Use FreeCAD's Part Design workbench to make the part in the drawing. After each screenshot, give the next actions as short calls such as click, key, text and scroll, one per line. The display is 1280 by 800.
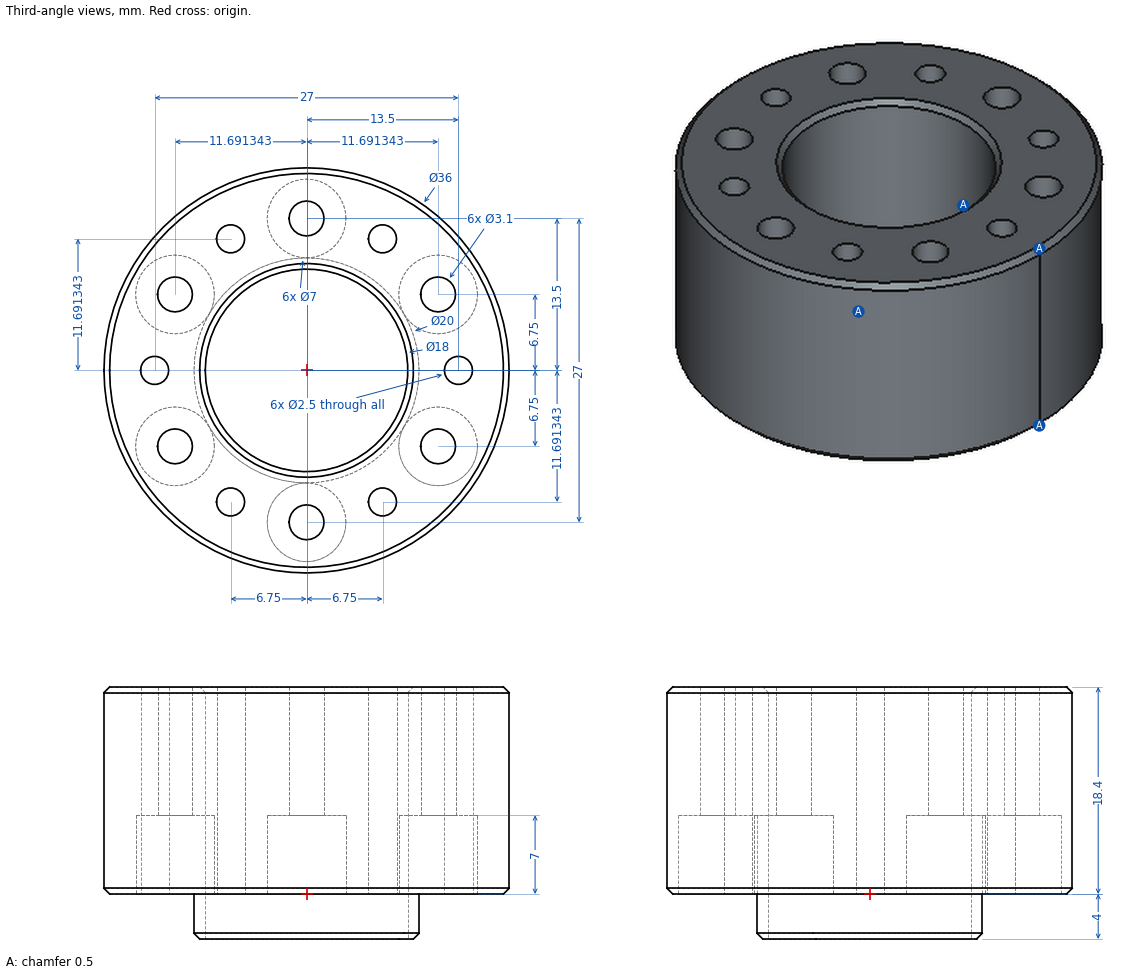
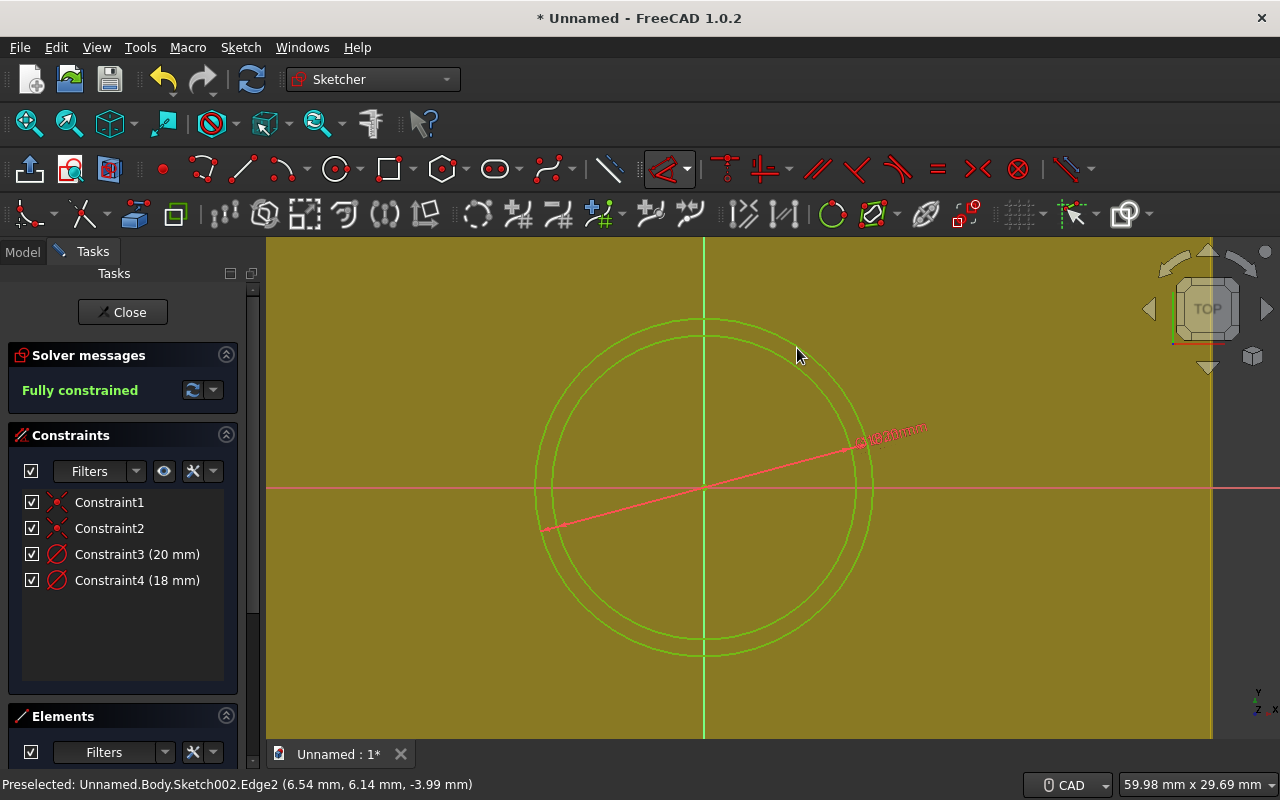
click(123, 312)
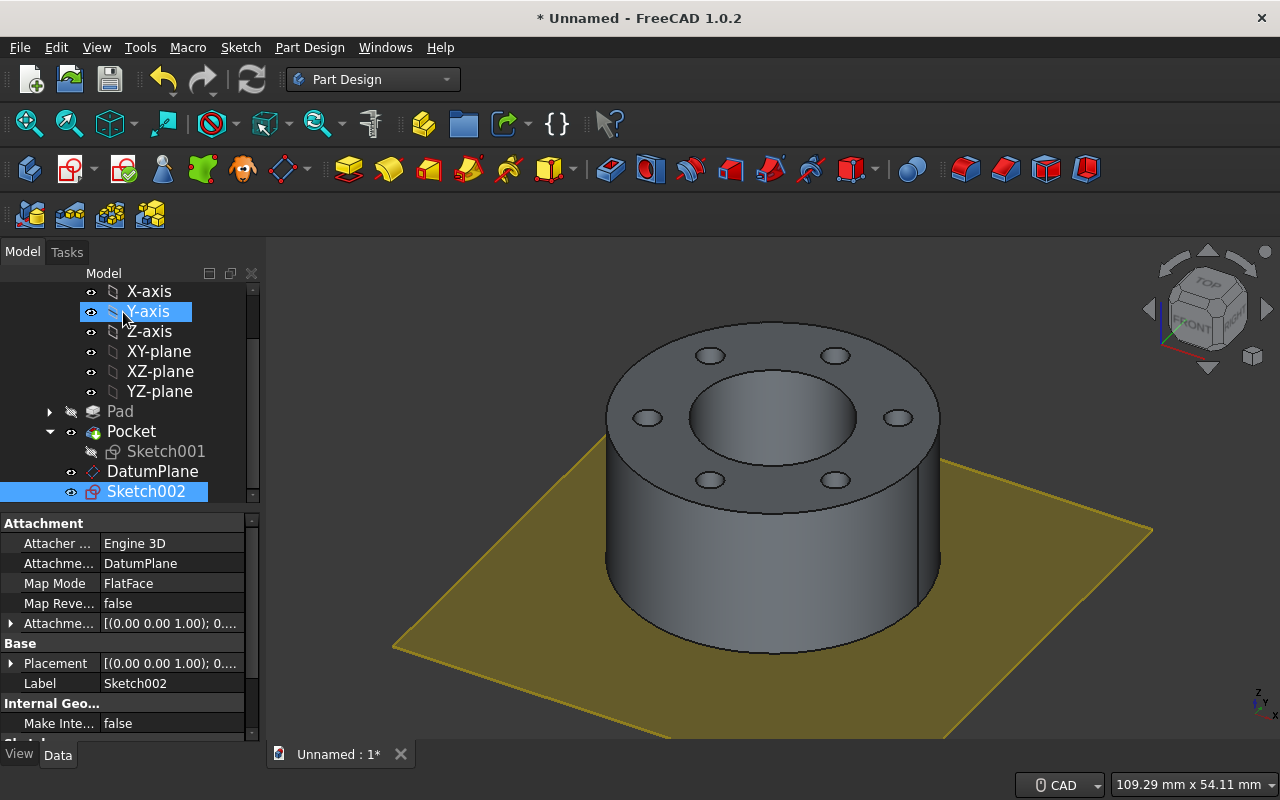
click(350, 170)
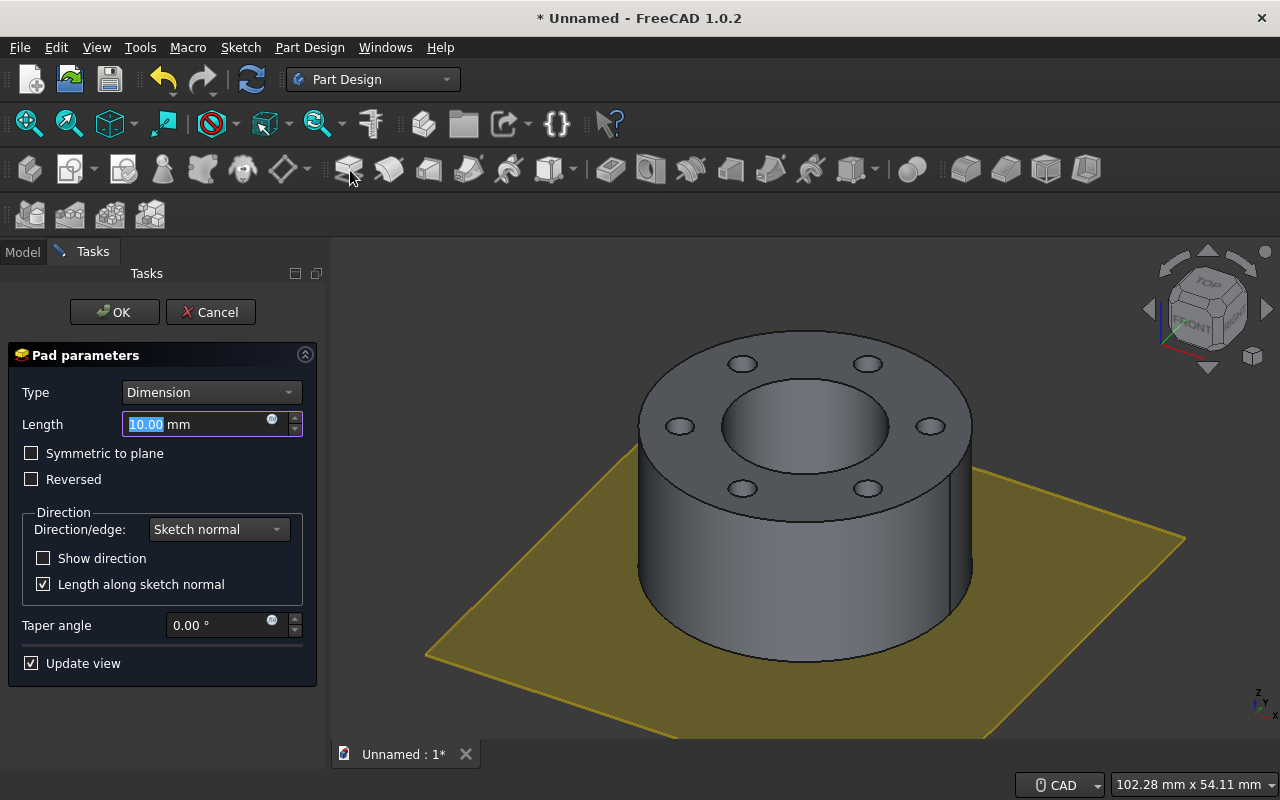
text(4)
key(Tab)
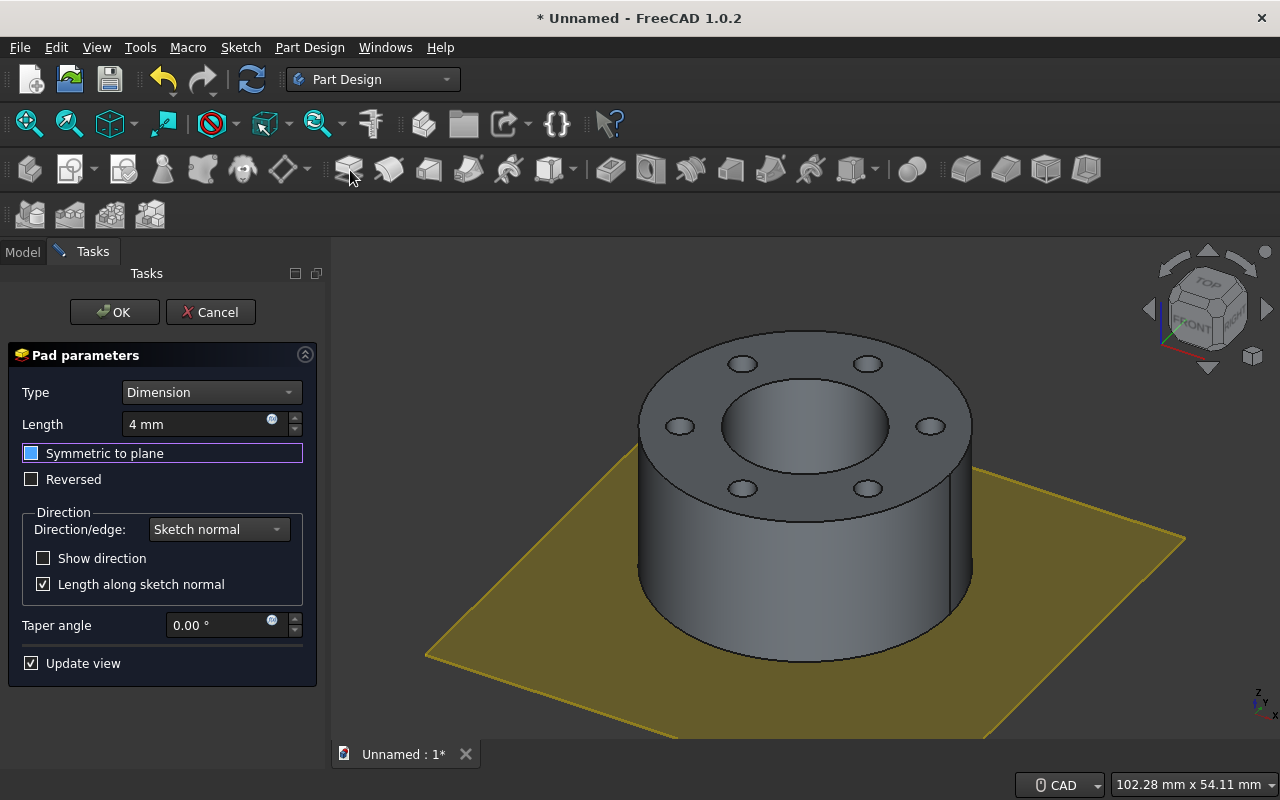
click(115, 312)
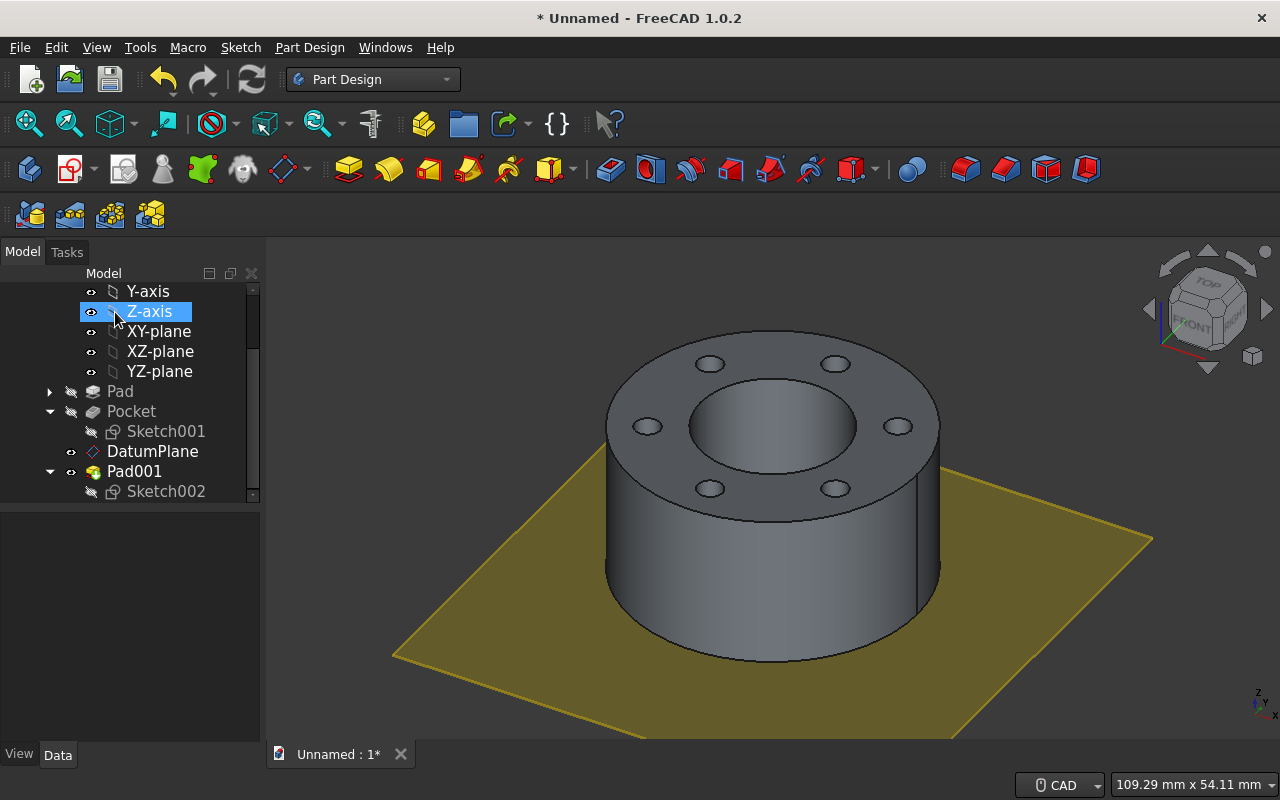
click(116, 452)
key(space)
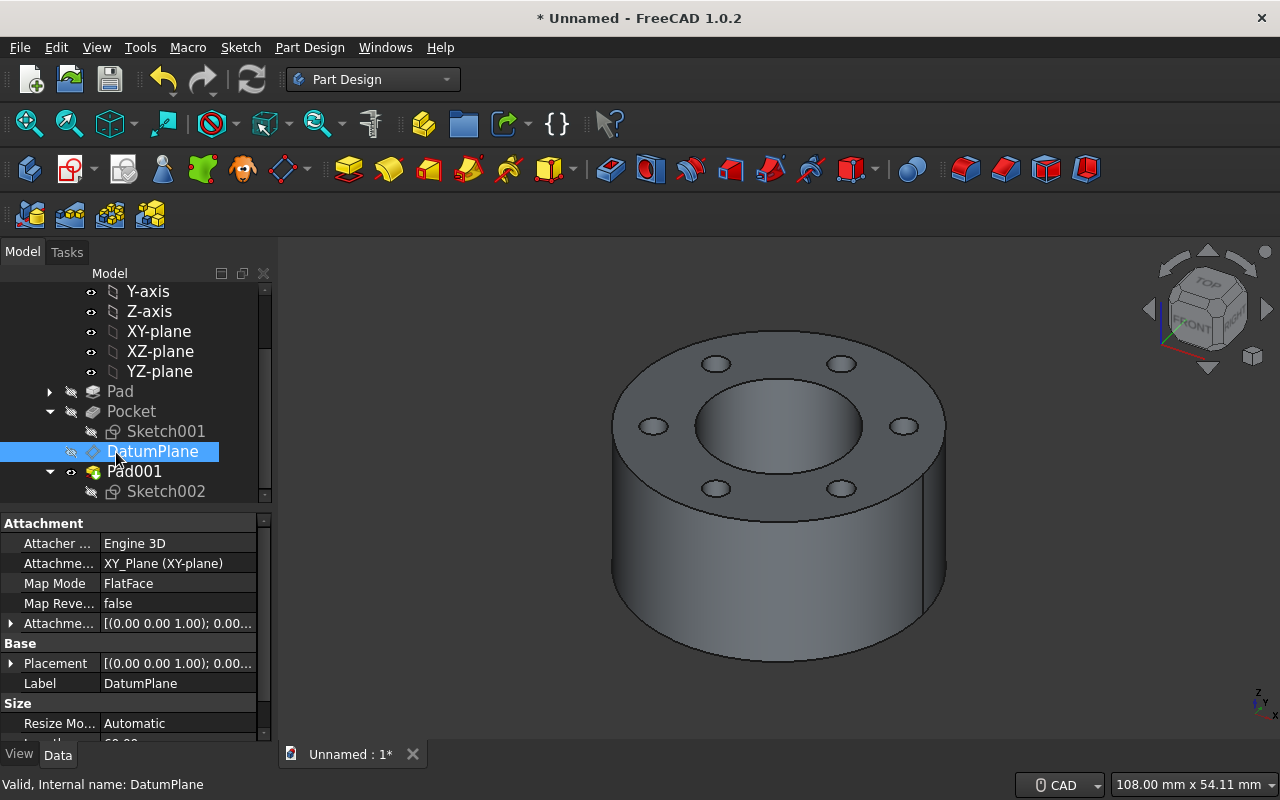
click(655, 384)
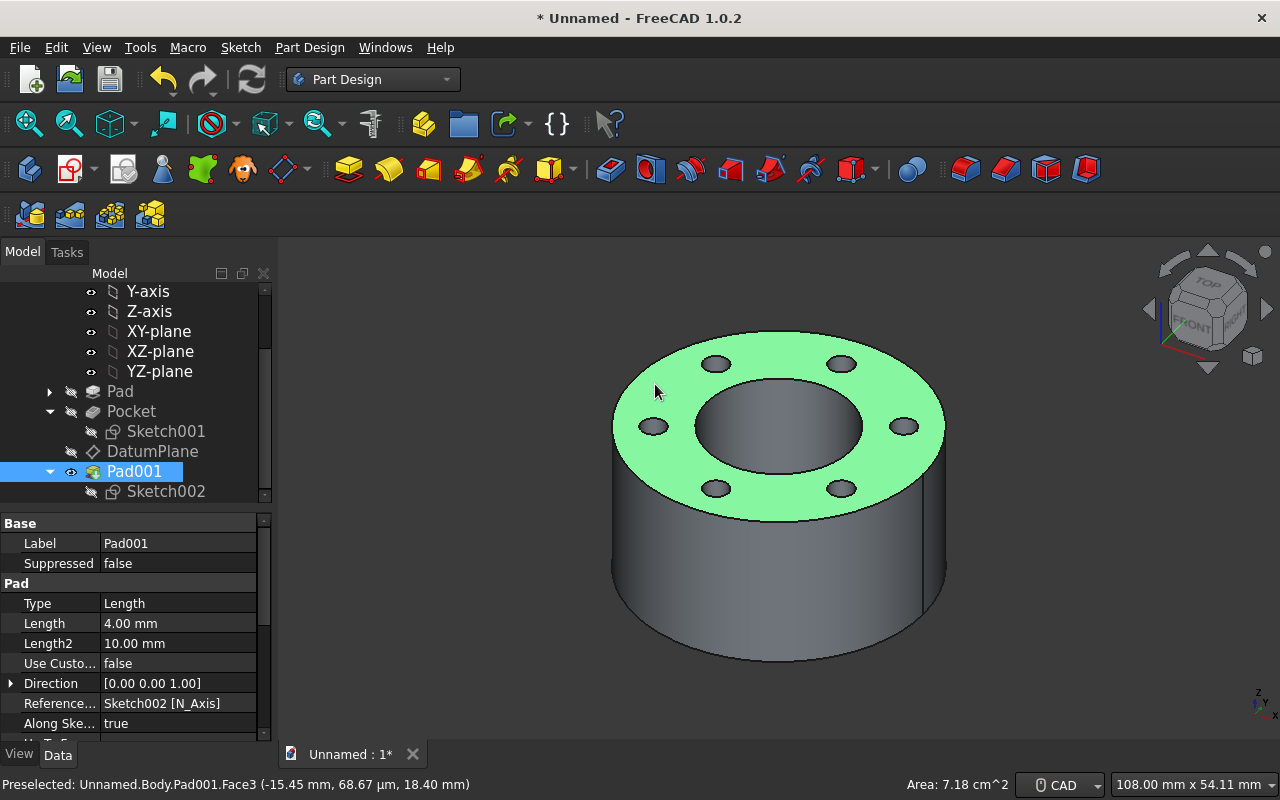
click(70, 170)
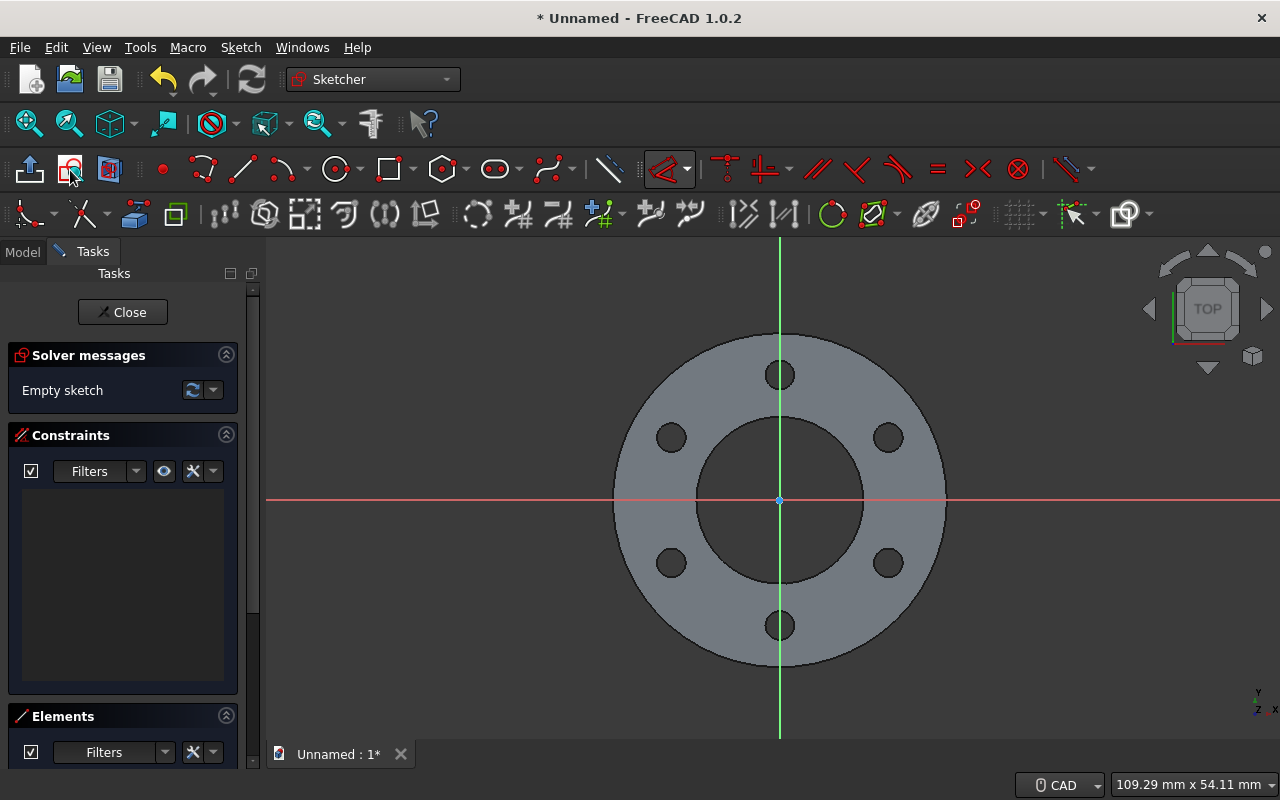
key(g)
key(c)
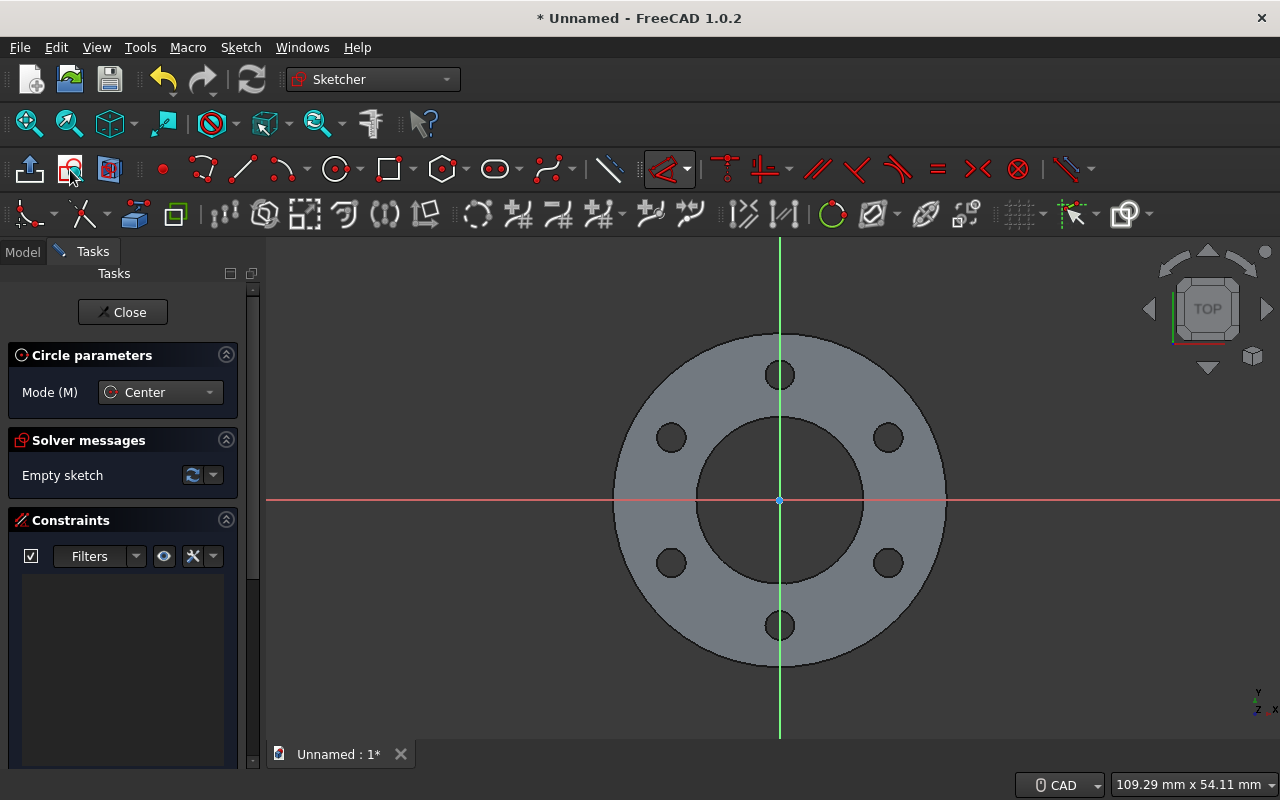
scroll(905, 500, up, 4)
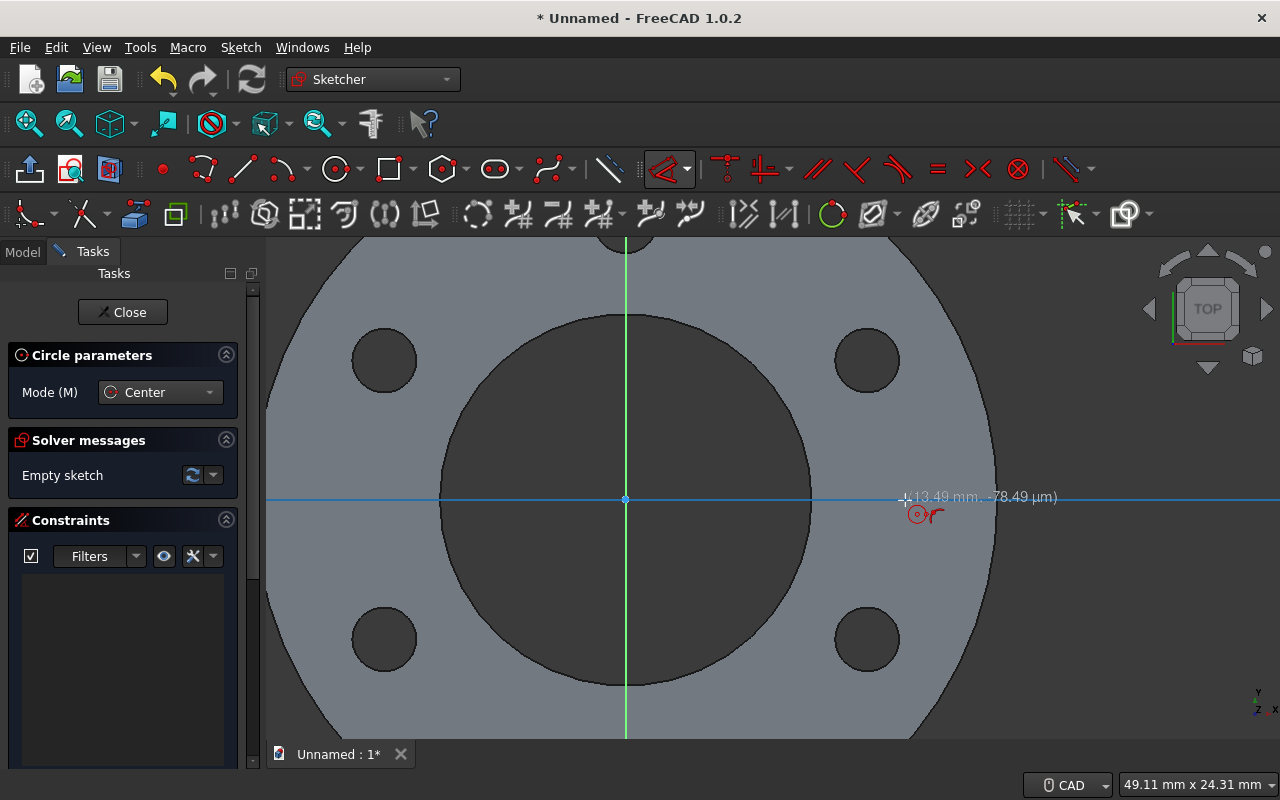
click(905, 500)
click(923, 482)